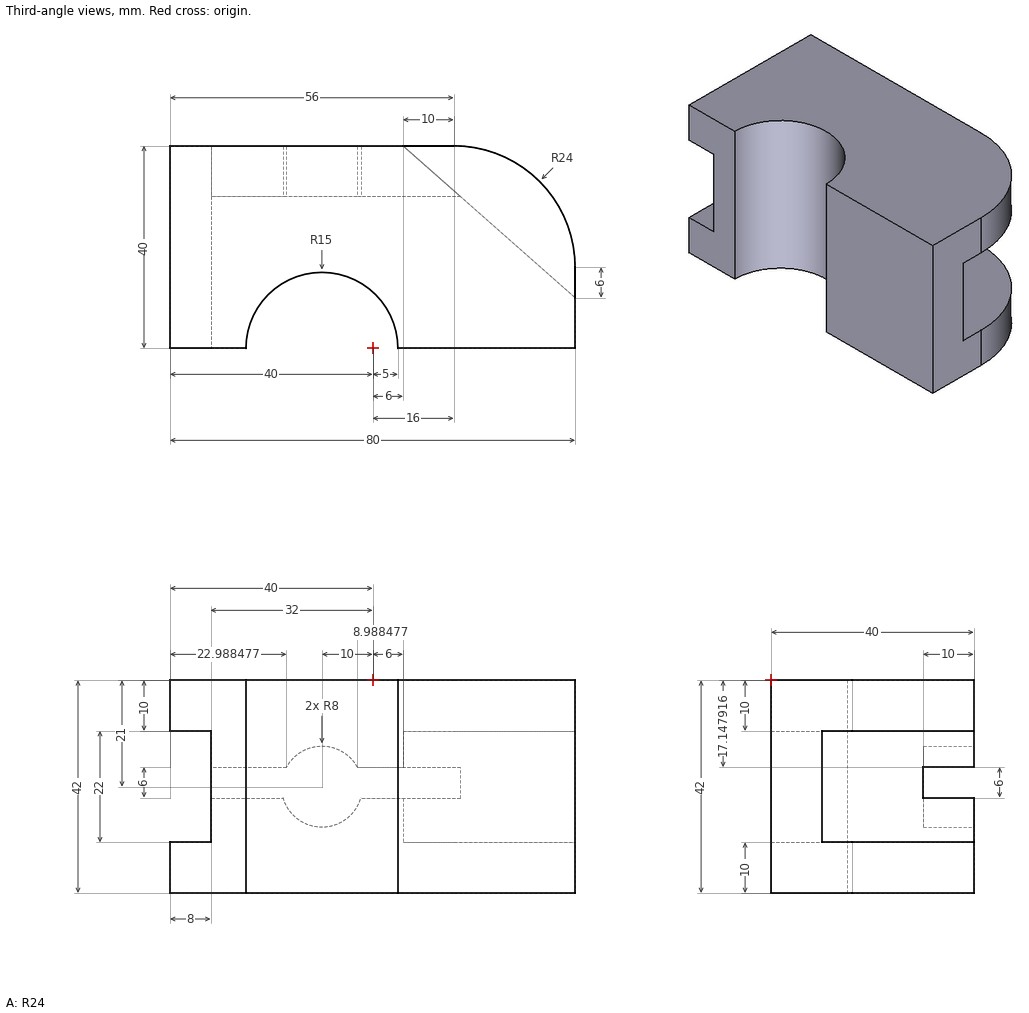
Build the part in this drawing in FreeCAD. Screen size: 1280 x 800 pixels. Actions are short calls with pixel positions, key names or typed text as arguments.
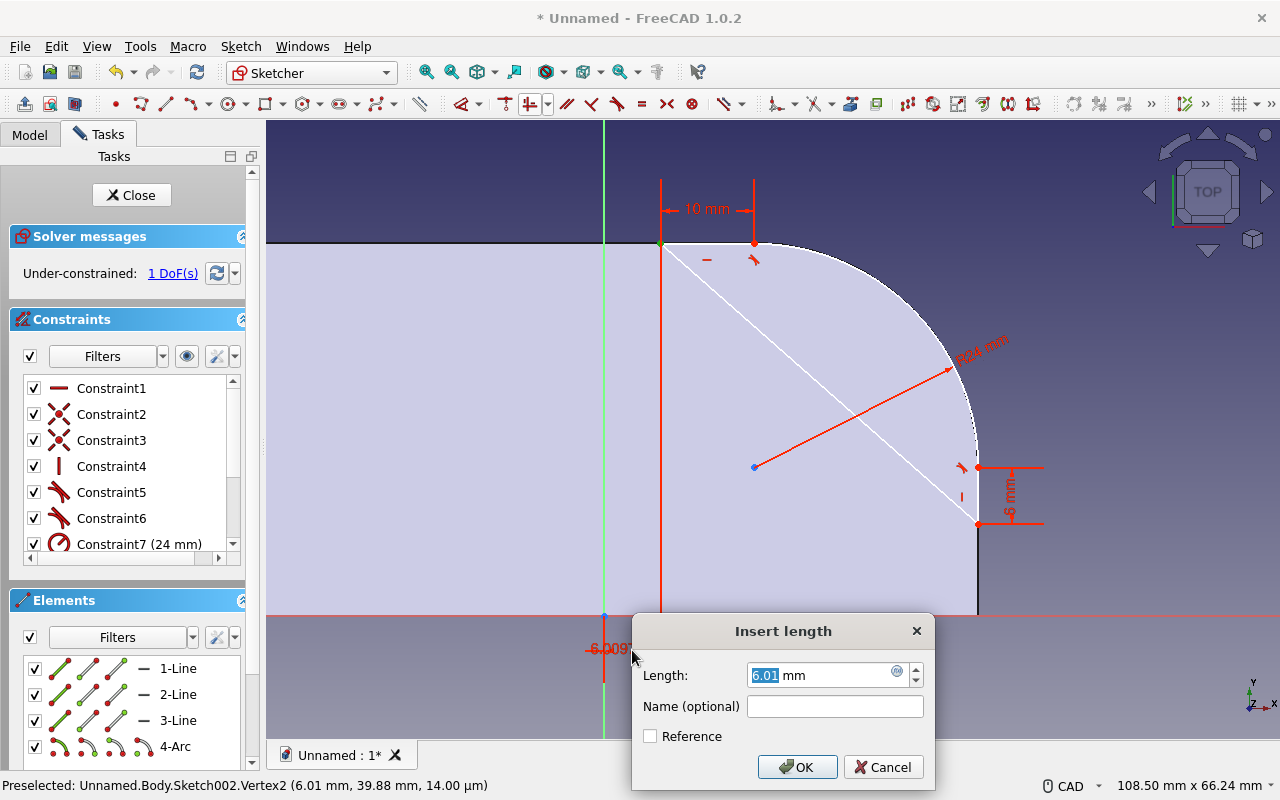
text(6)
key(Return)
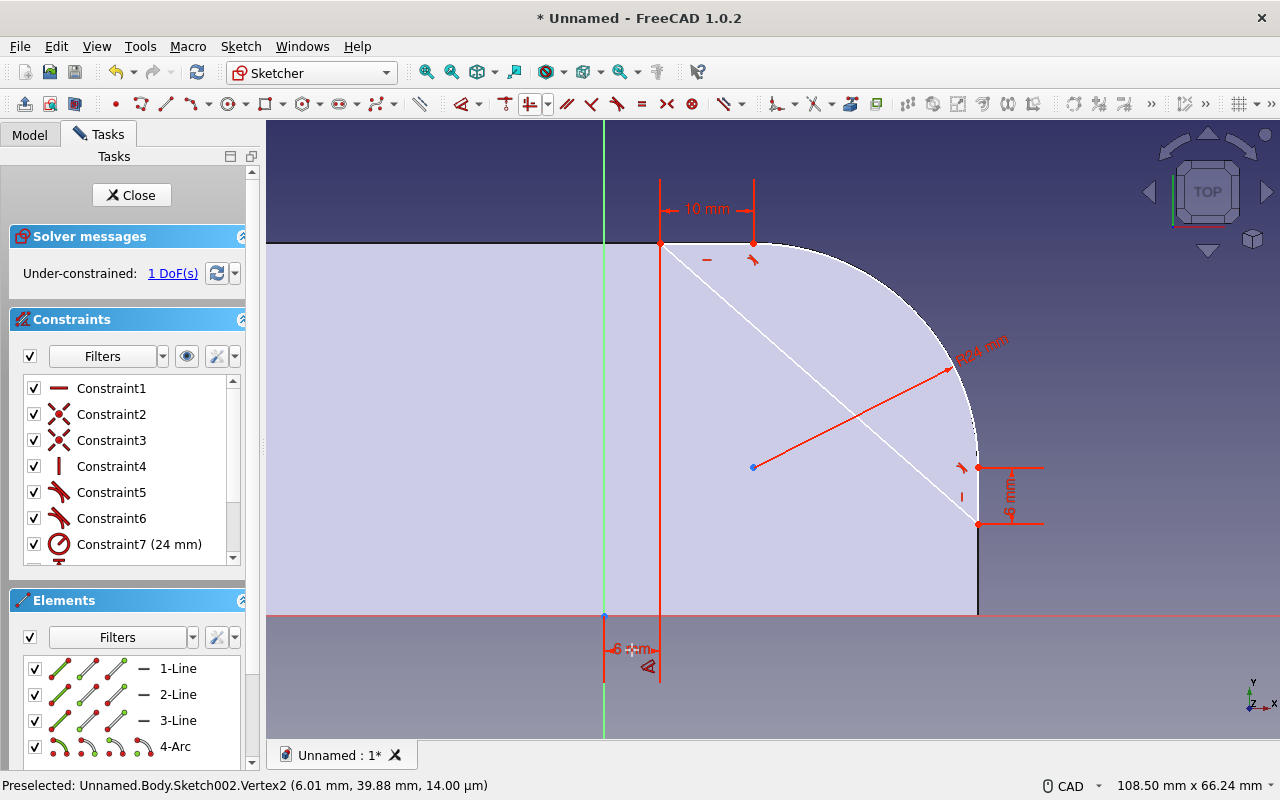
click(754, 244)
click(570, 430)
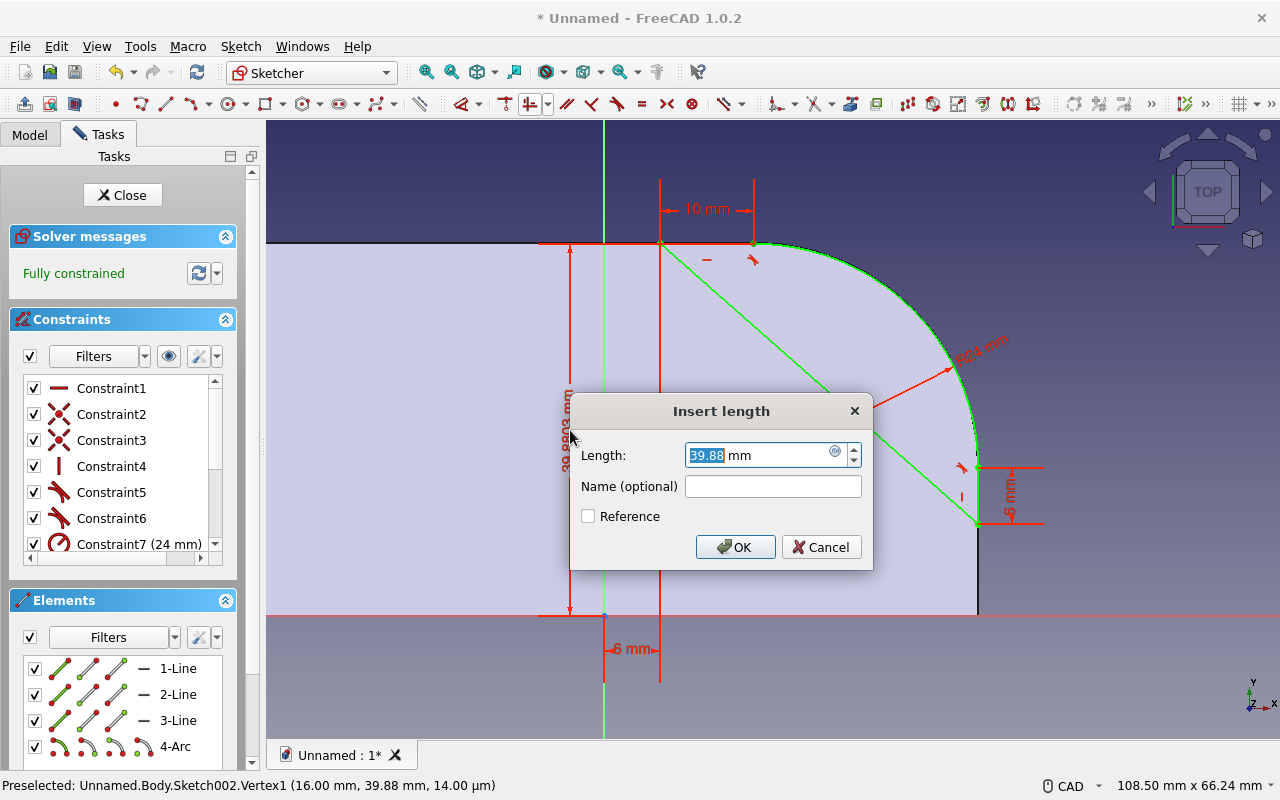
text(40)
key(Return)
key(Escape)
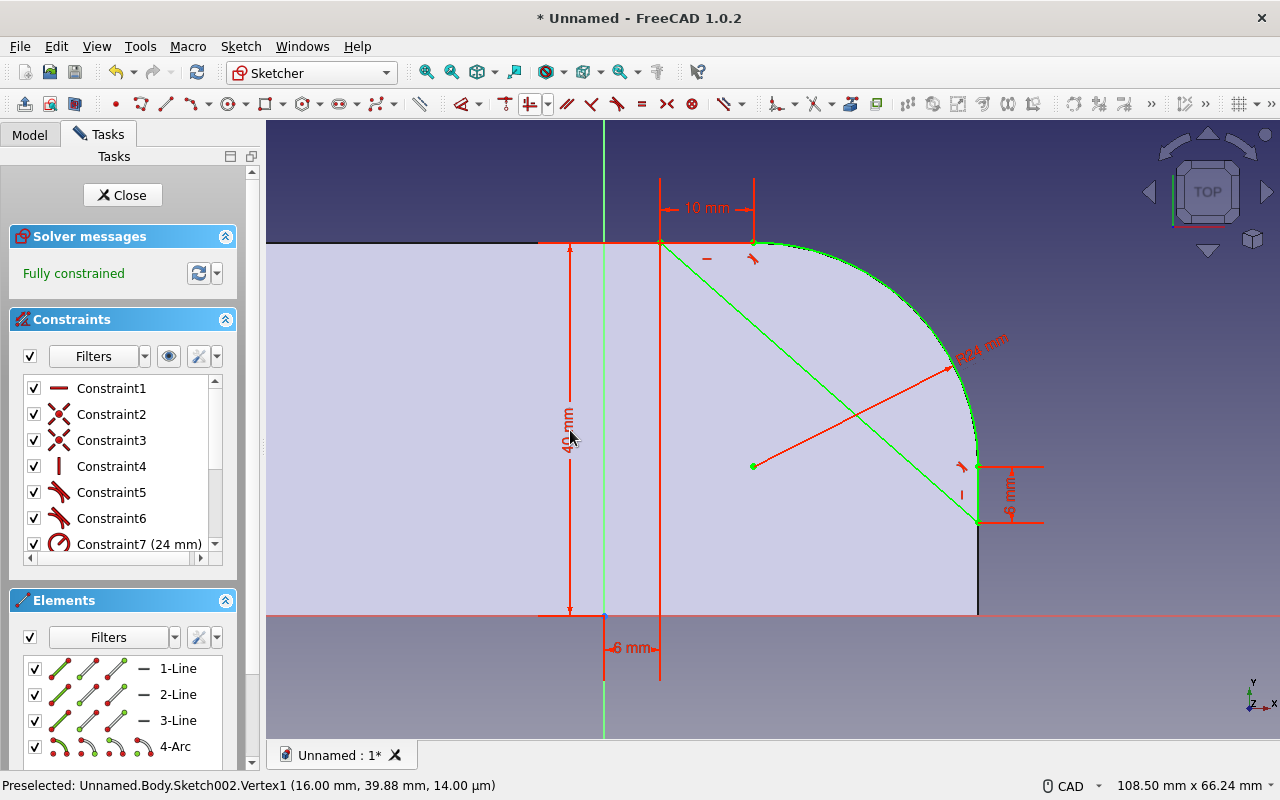
click(123, 195)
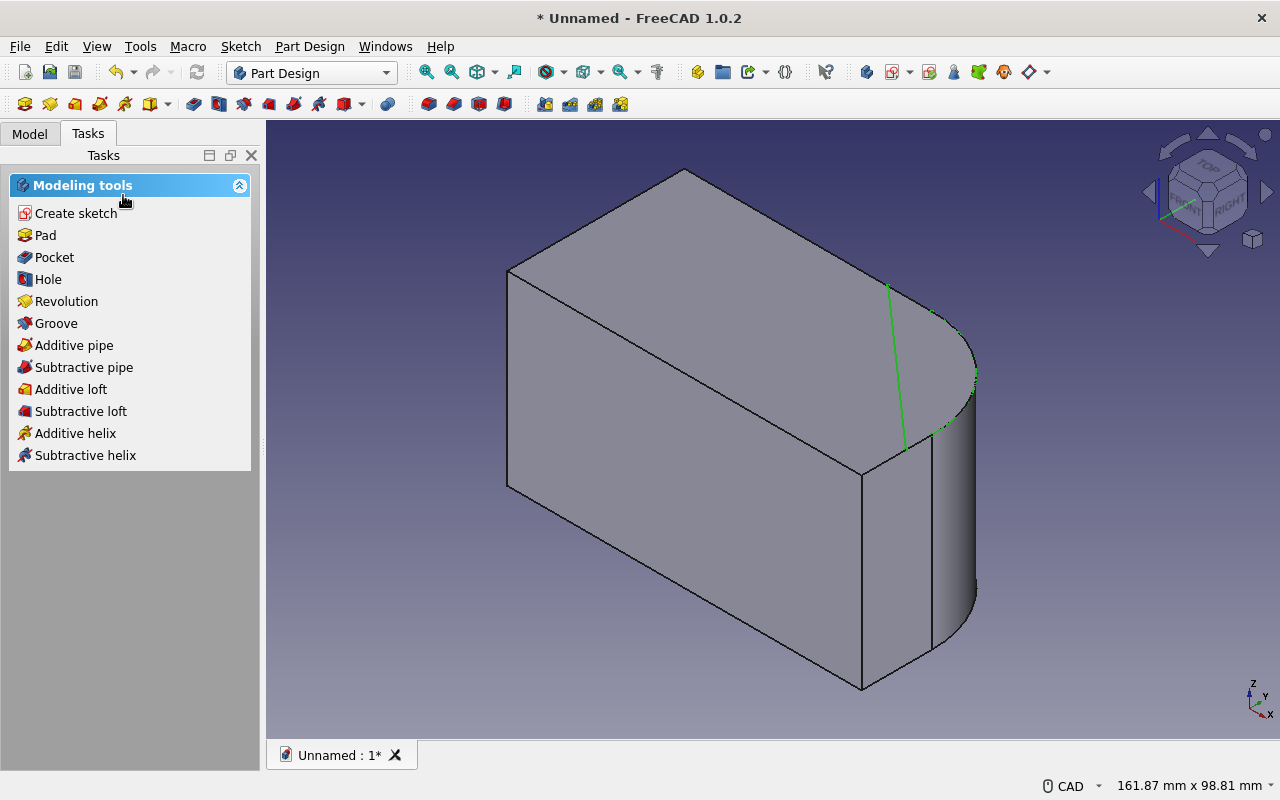
click(194, 104)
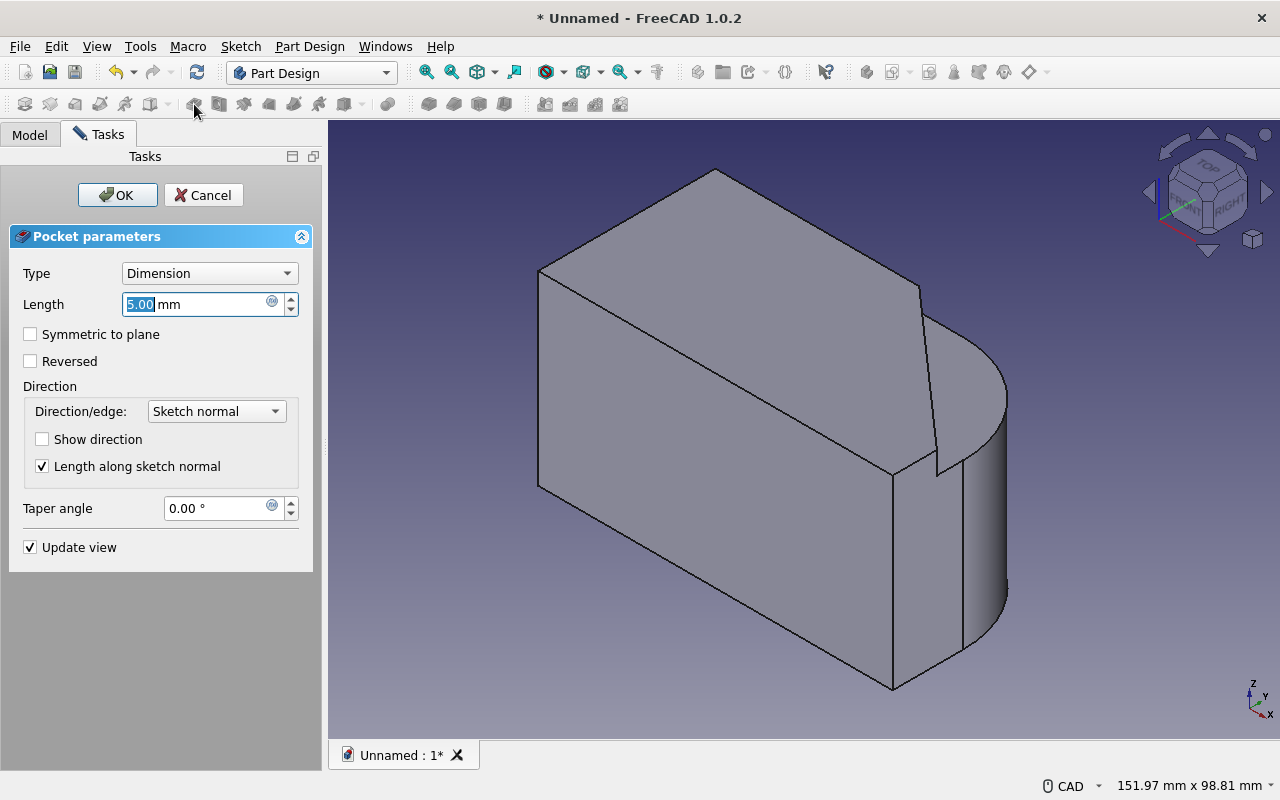
text(42)
key(Tab)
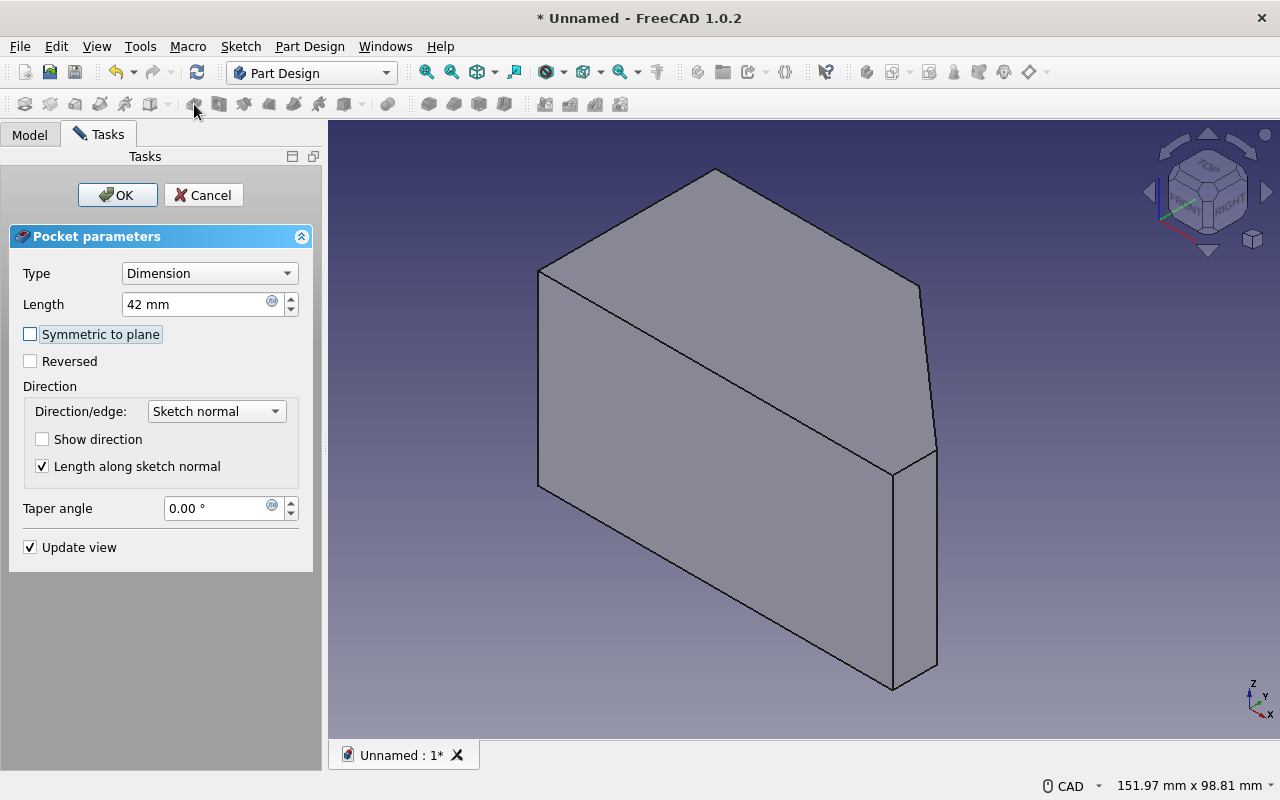
click(118, 195)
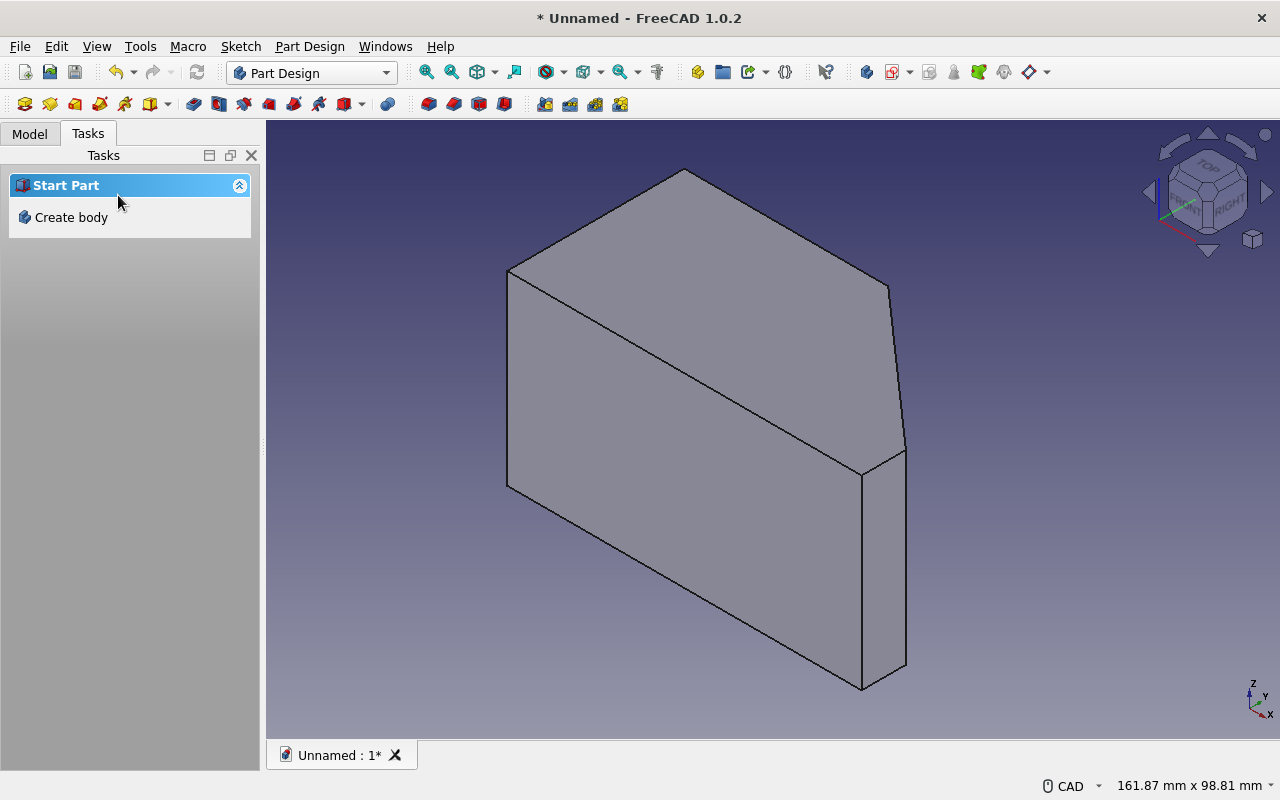
key(6)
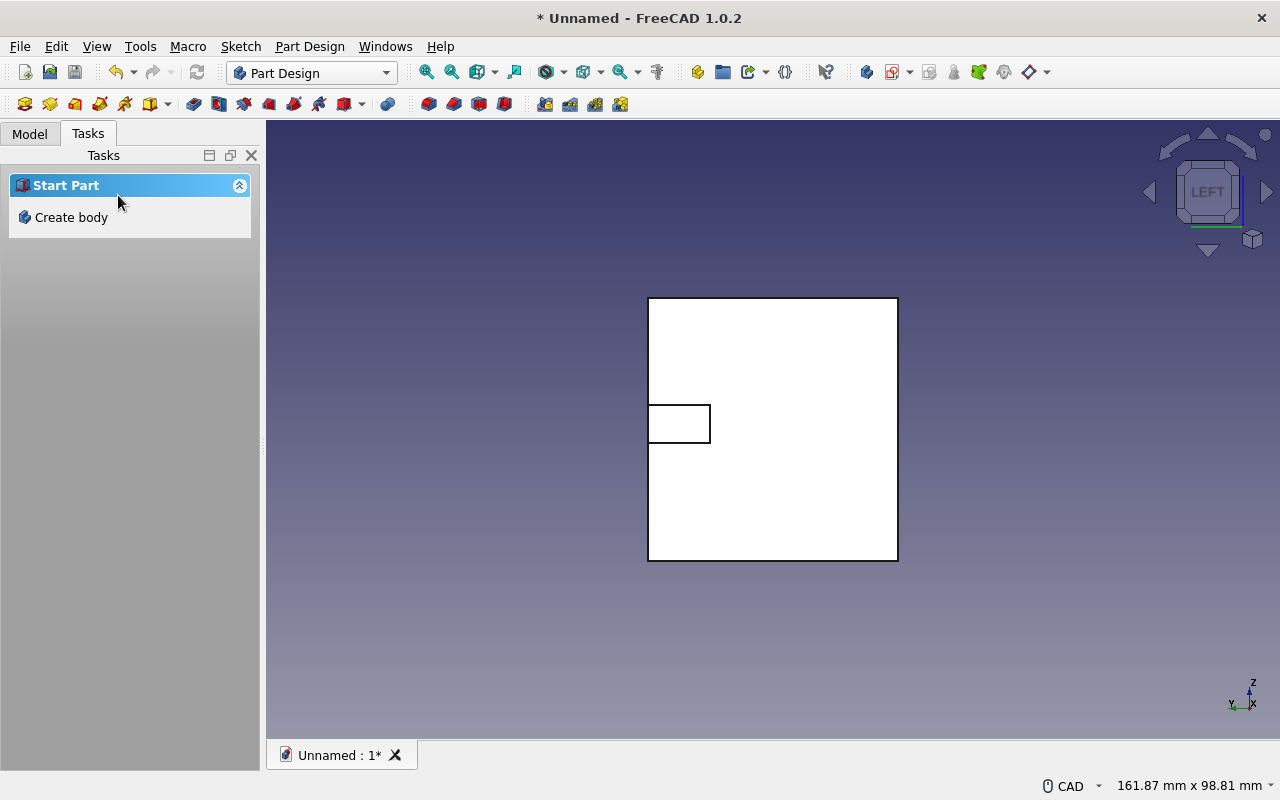
key(v)
key(f)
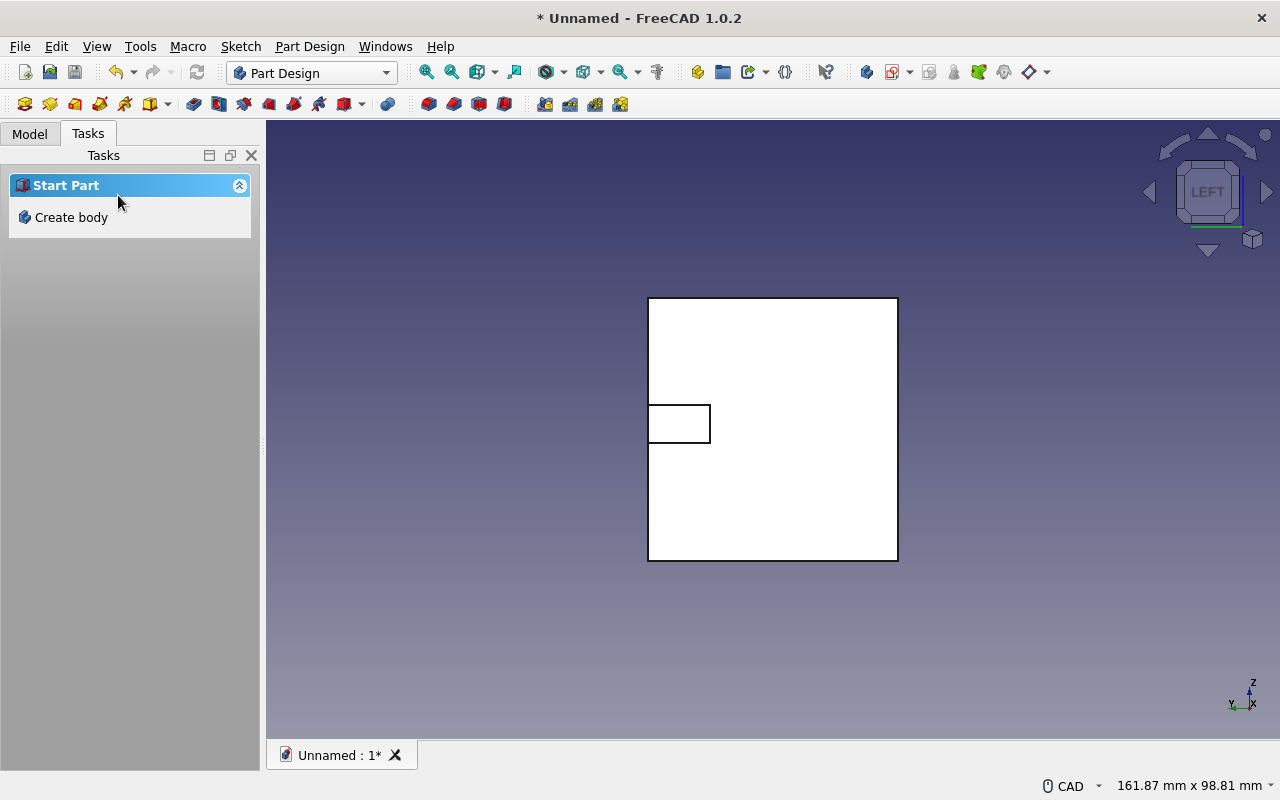
click(670, 423)